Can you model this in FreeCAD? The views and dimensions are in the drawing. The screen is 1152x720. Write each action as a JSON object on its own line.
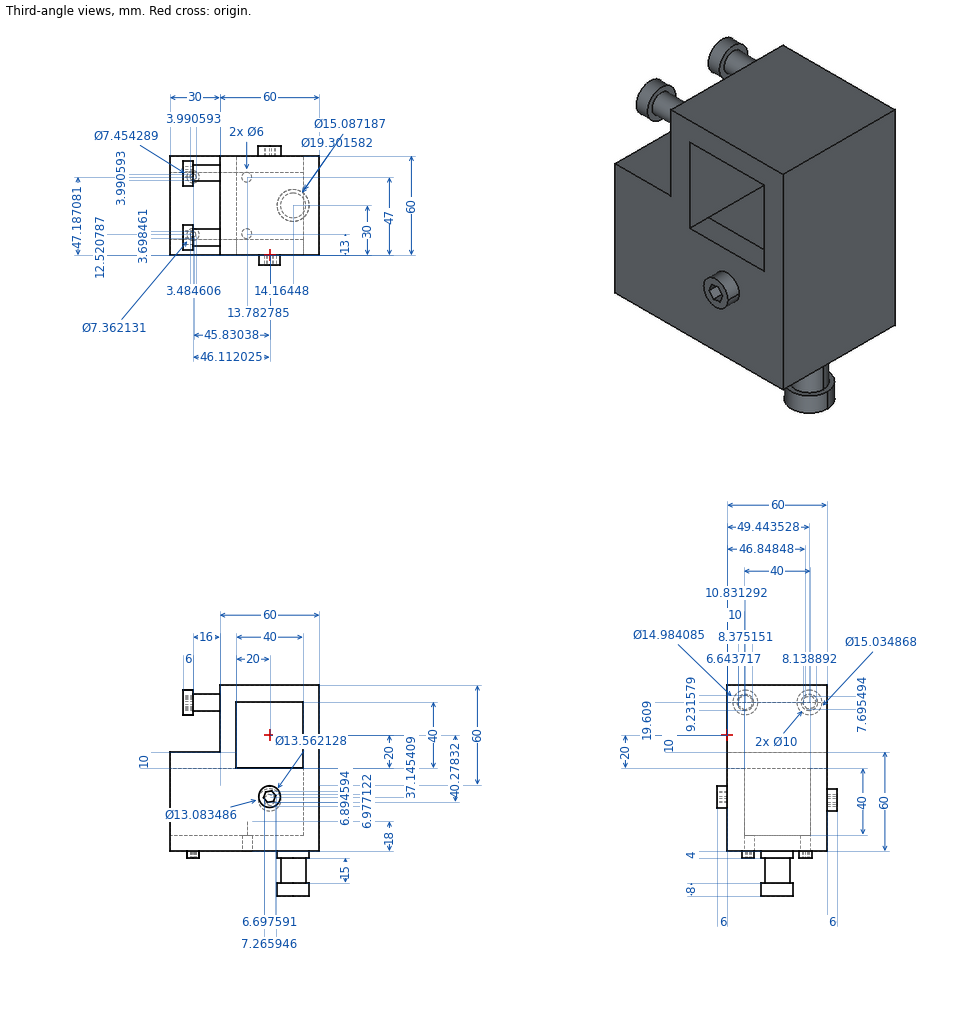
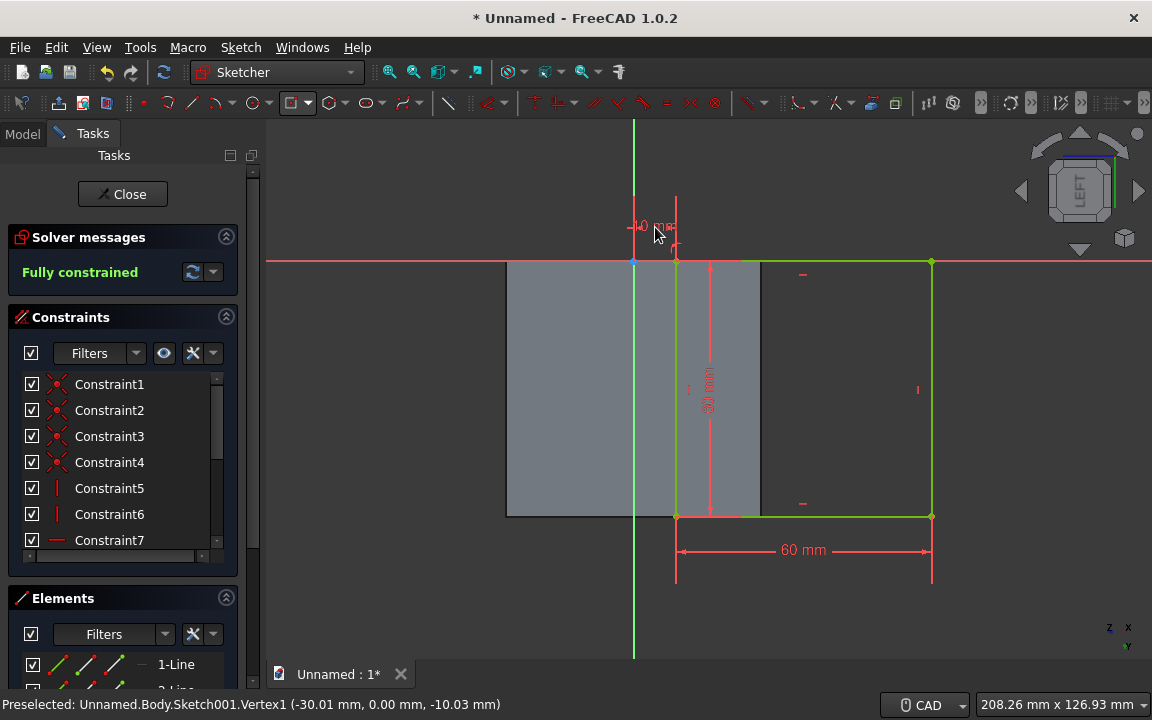
{"action": "left_click", "coordinate": [123, 194]}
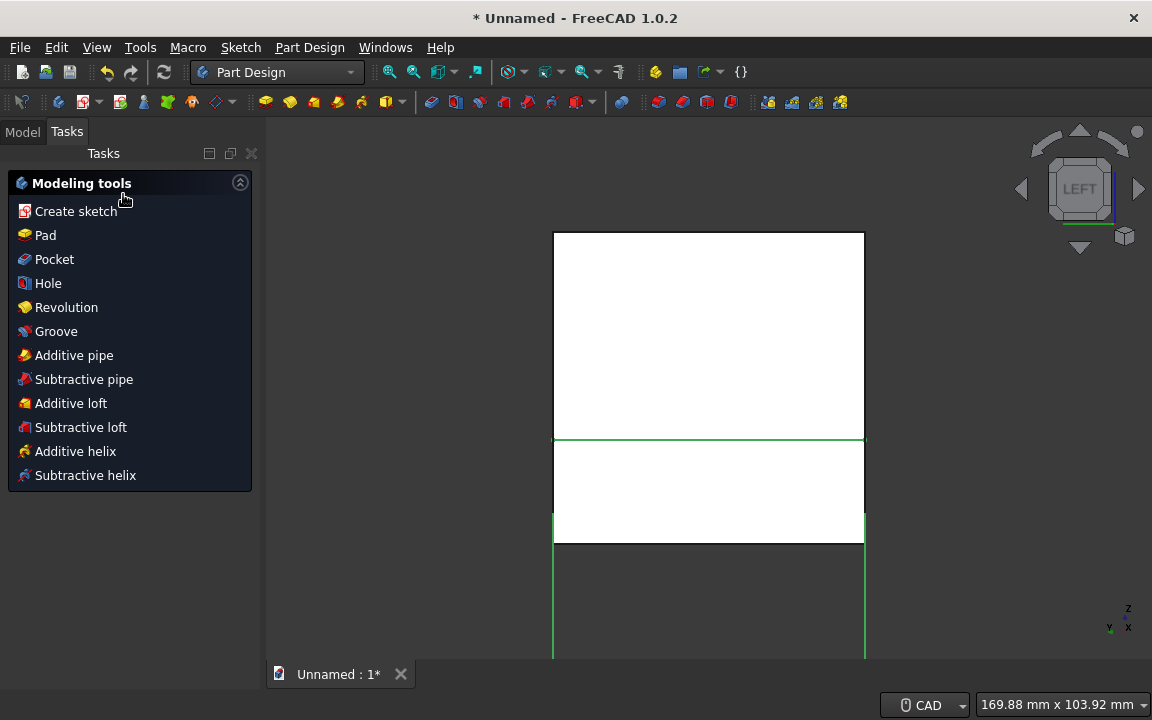
{"action": "left_click", "coordinate": [266, 102]}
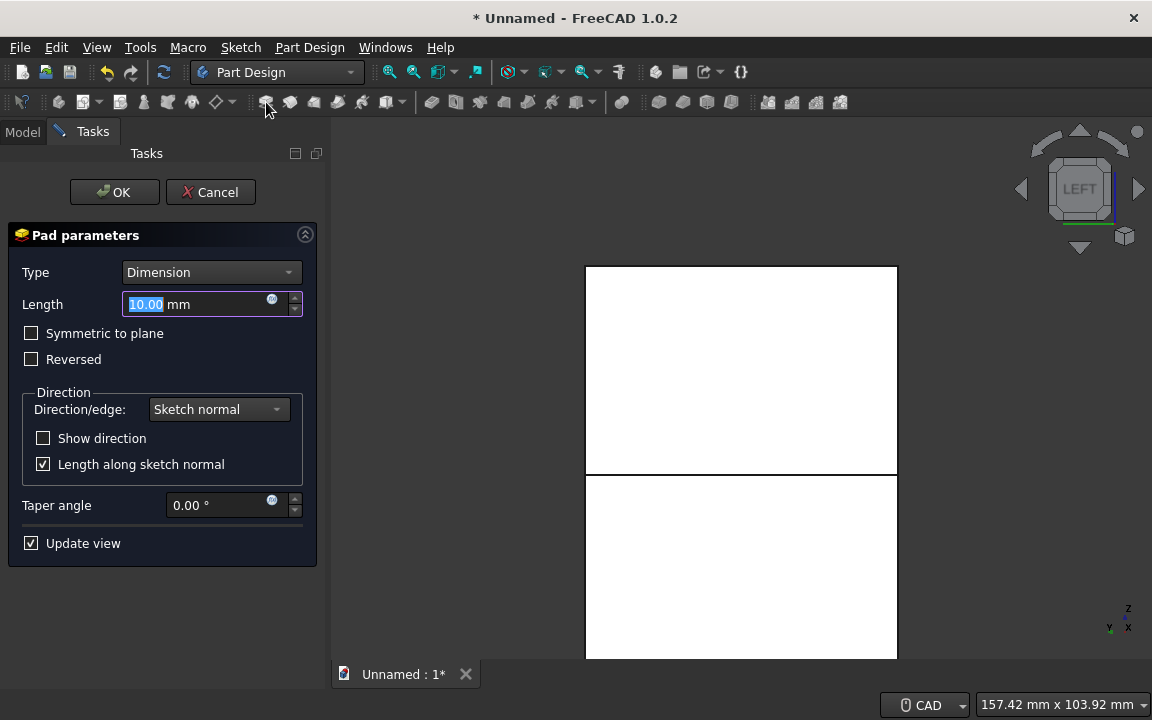
{"action": "left_click", "coordinate": [212, 272]}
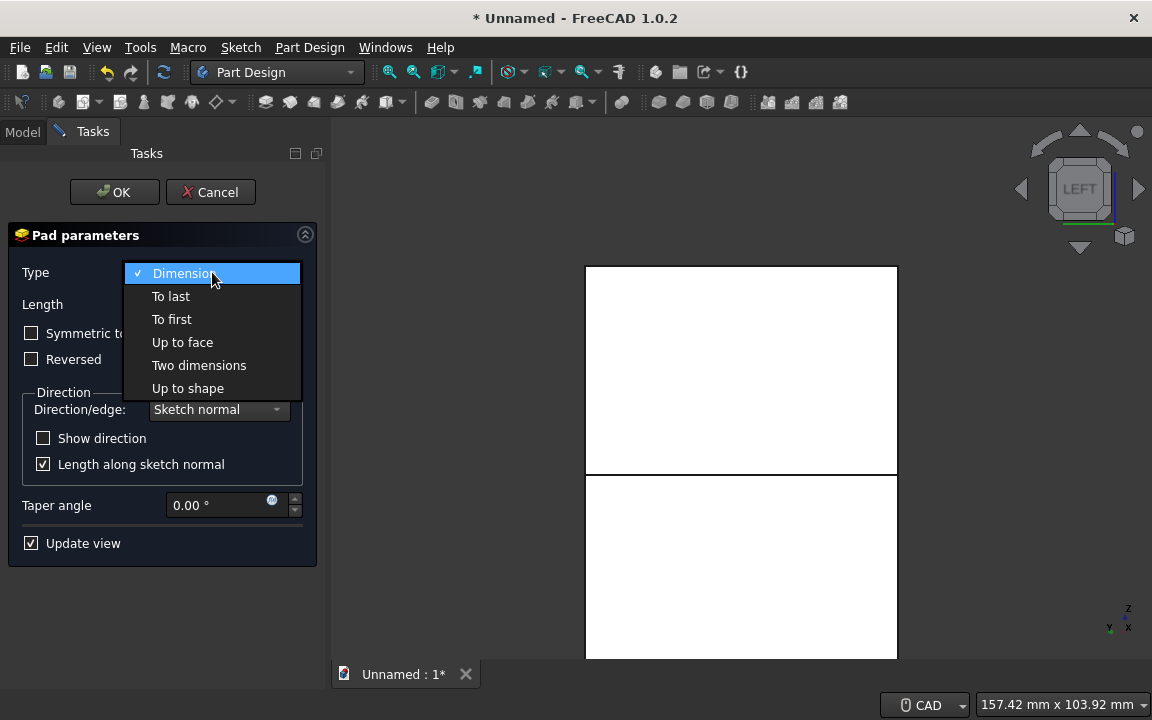
{"action": "left_click", "coordinate": [212, 366]}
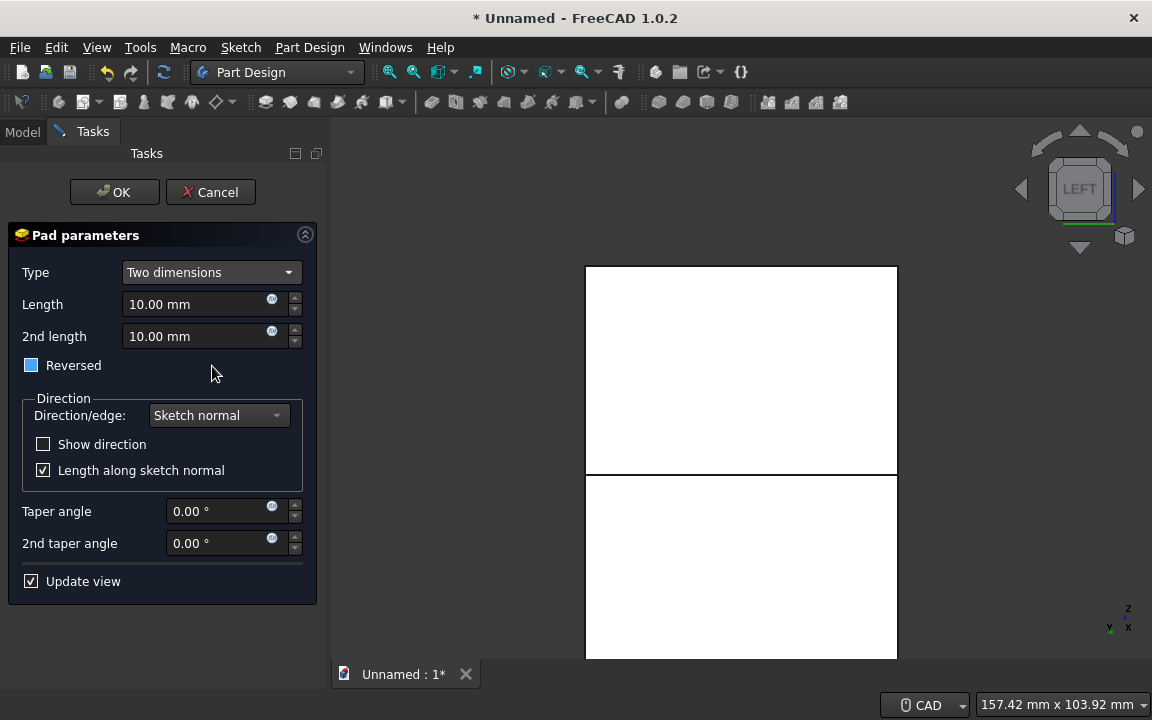
{"action": "triple_click", "coordinate": [204, 304]}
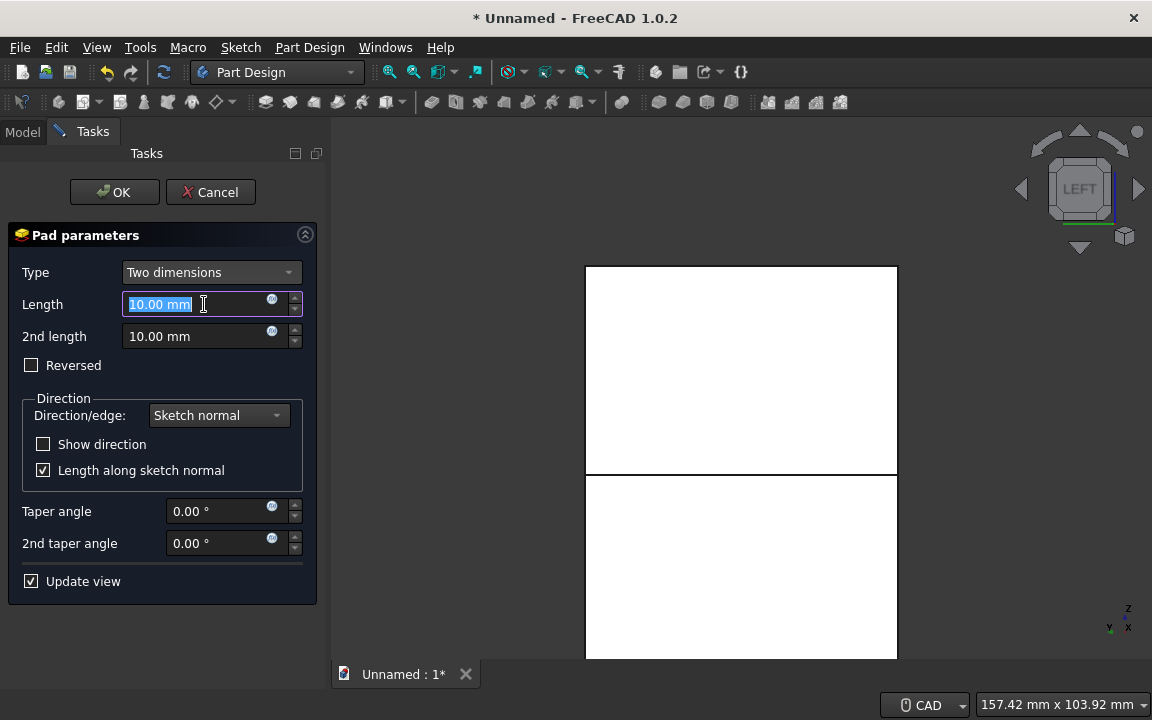
{"action": "type", "text": "30"}
{"action": "key", "text": "Tab"}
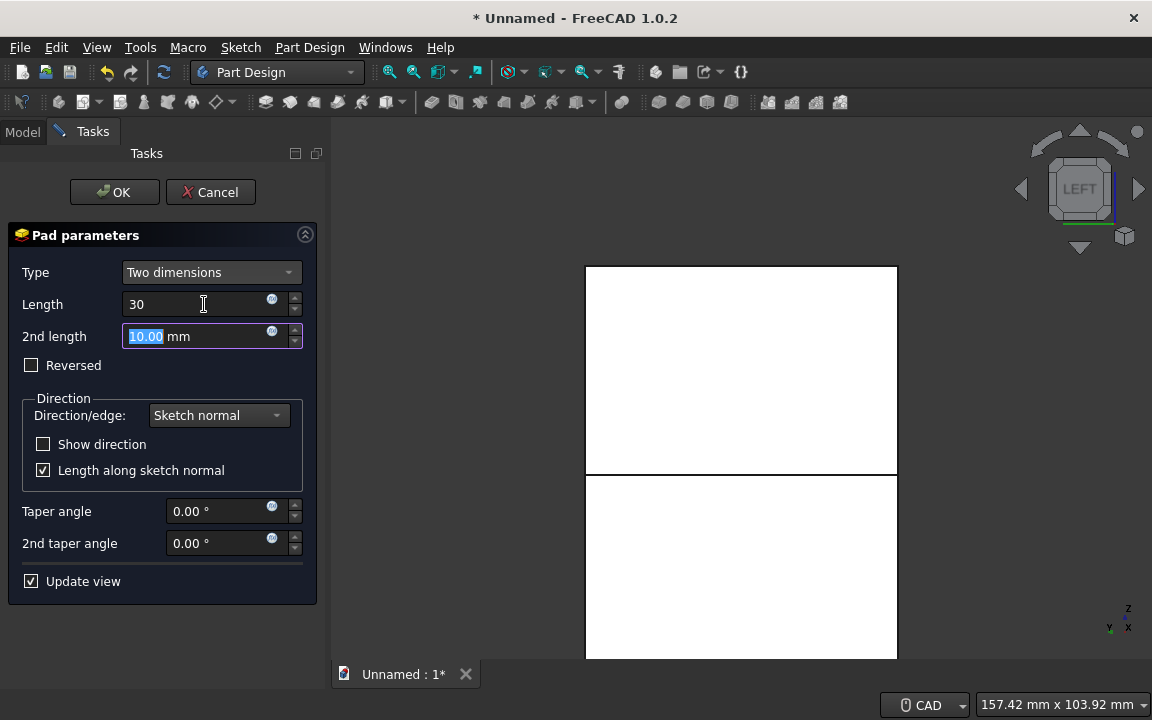
{"action": "type", "text": "60"}
{"action": "key", "text": "Tab"}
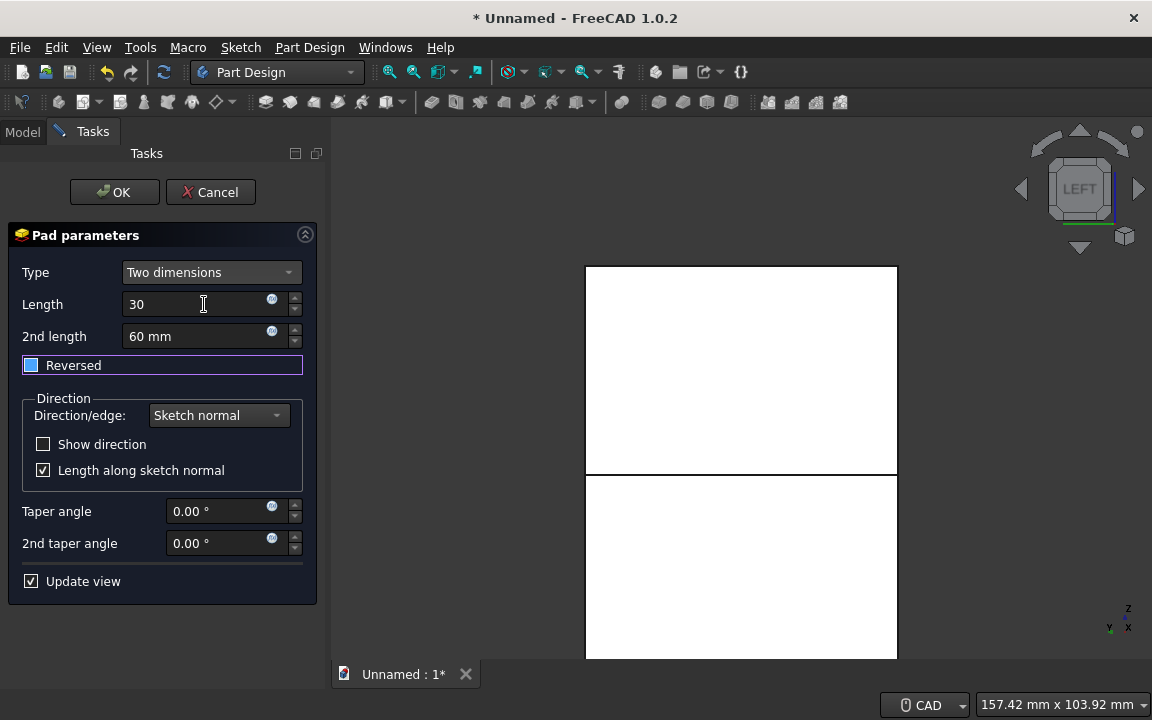
{"action": "left_click", "coordinate": [115, 192]}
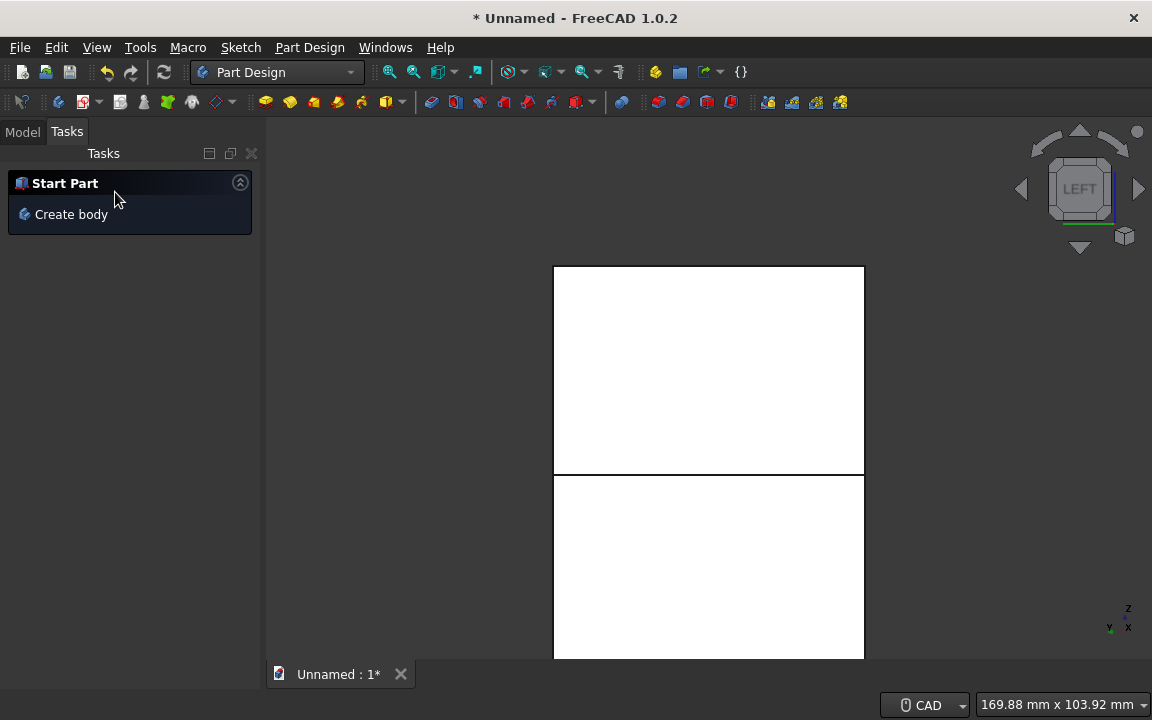
{"action": "left_click", "coordinate": [390, 72]}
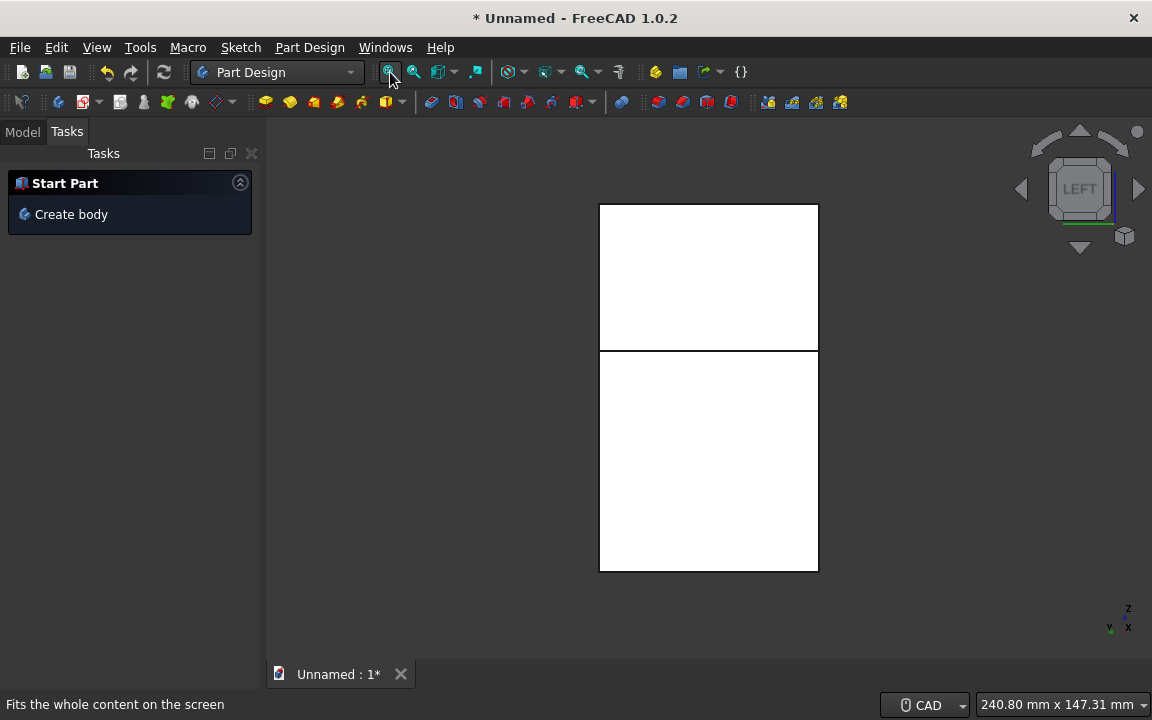
{"action": "left_click", "coordinate": [741, 277]}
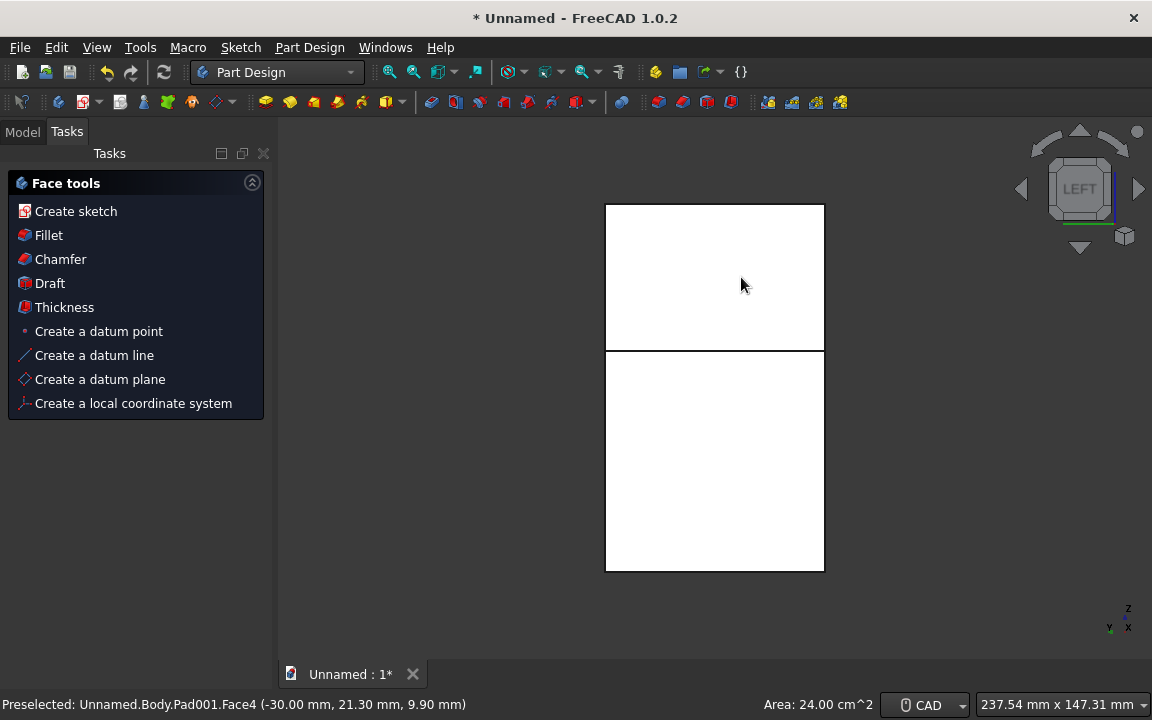
{"action": "left_click", "coordinate": [84, 102]}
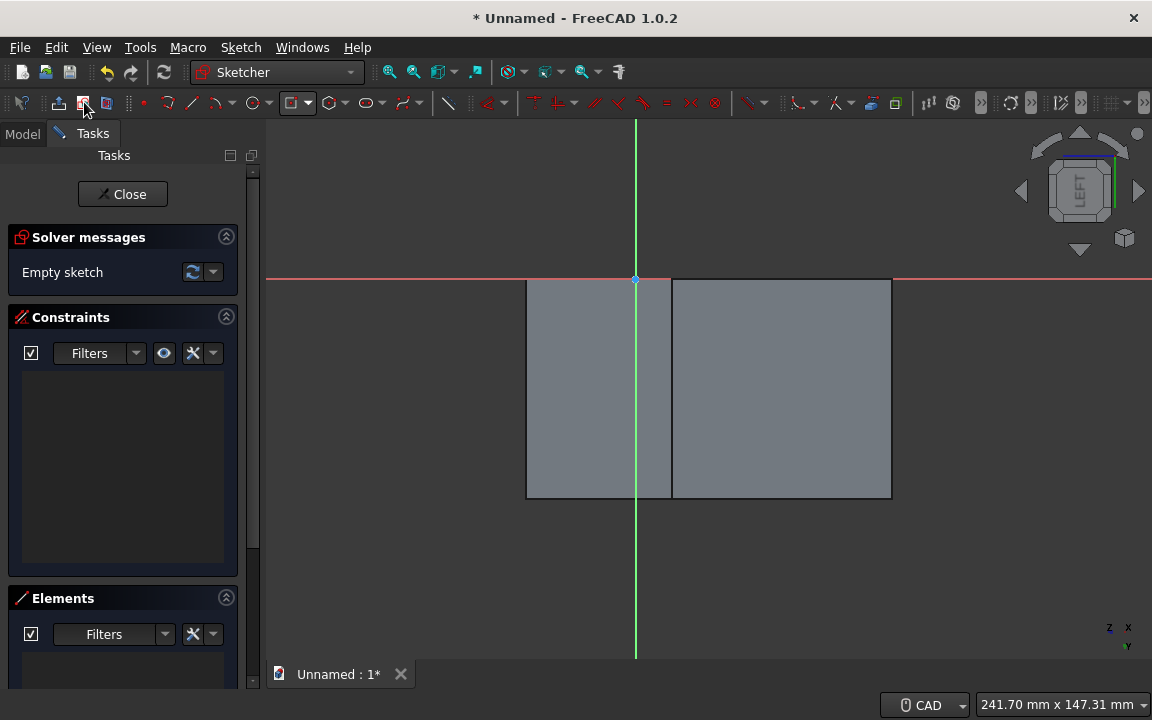
{"action": "left_click", "coordinate": [108, 104]}